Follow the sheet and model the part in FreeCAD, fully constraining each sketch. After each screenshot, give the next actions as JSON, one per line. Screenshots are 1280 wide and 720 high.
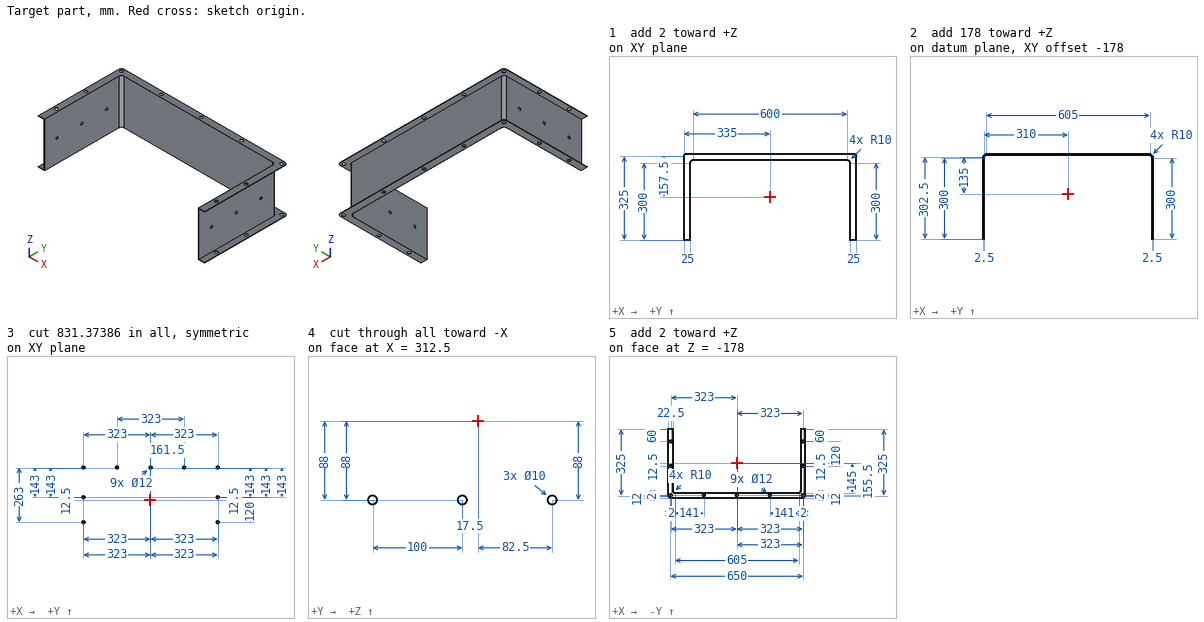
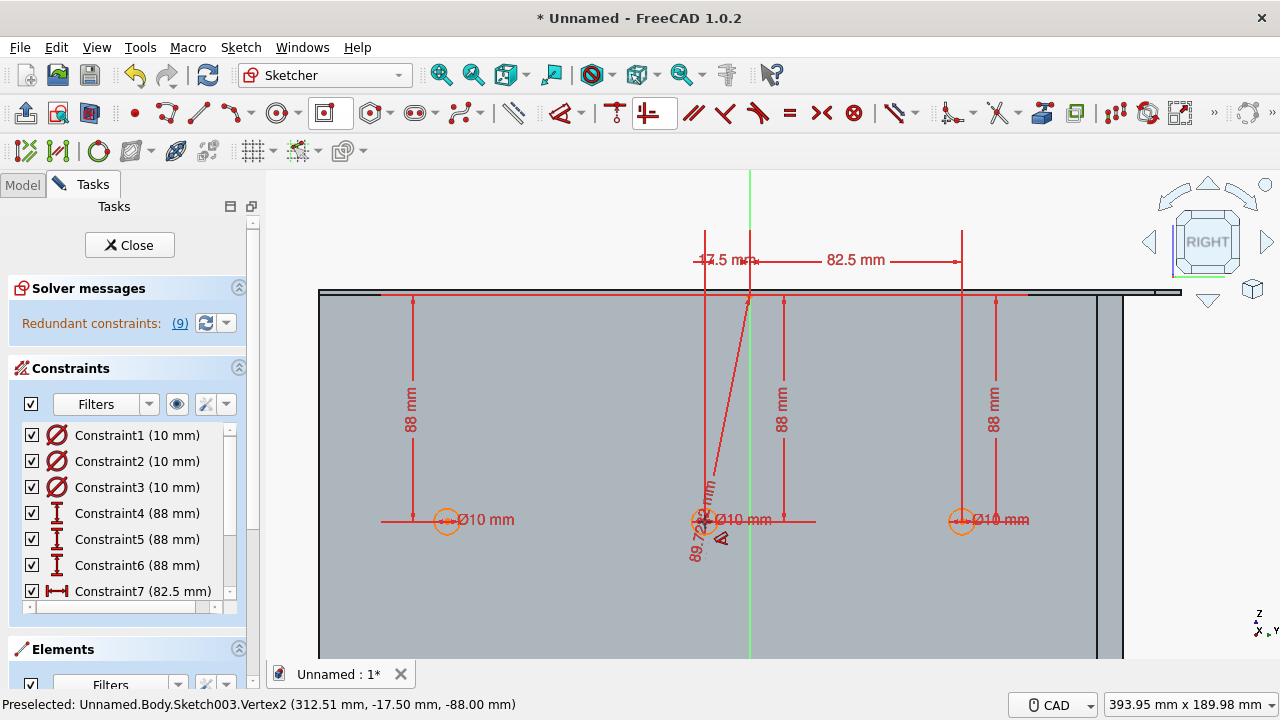
{"action": "left_click", "coordinate": [447, 522]}
{"action": "left_click", "coordinate": [576, 556]}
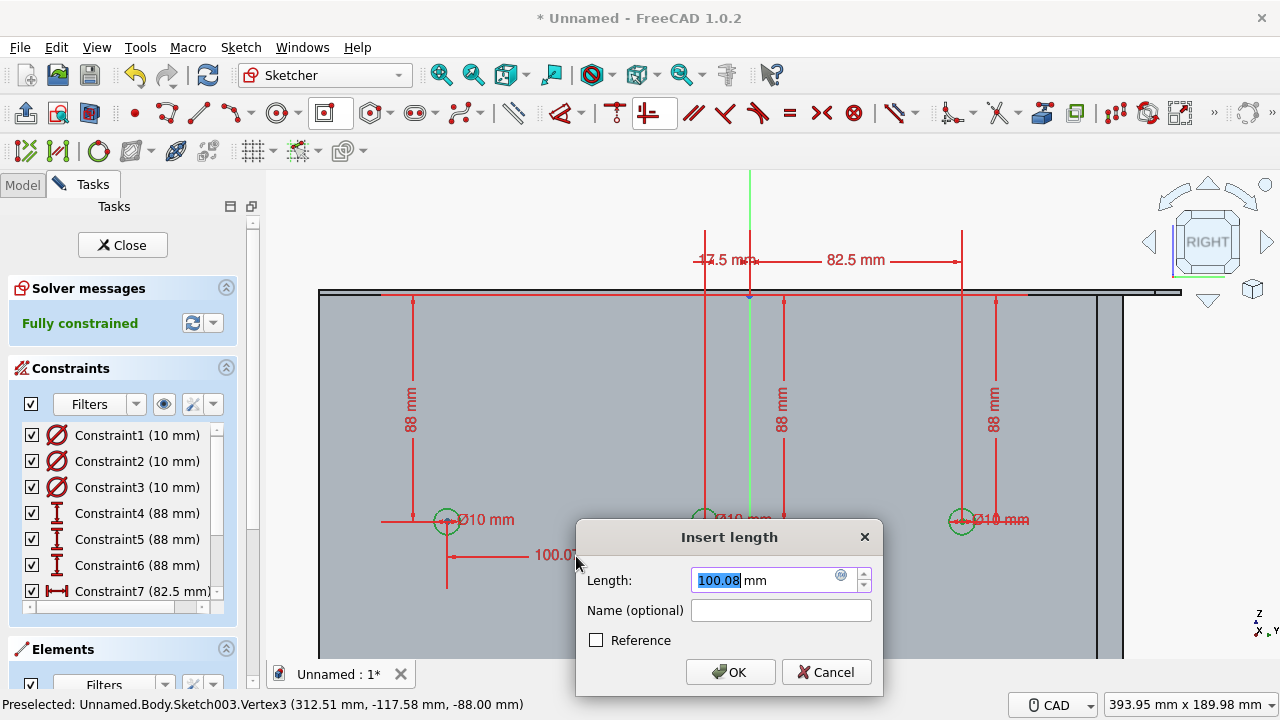
{"action": "type", "text": "100"}
{"action": "key", "text": "Return"}
{"action": "key", "text": "Escape"}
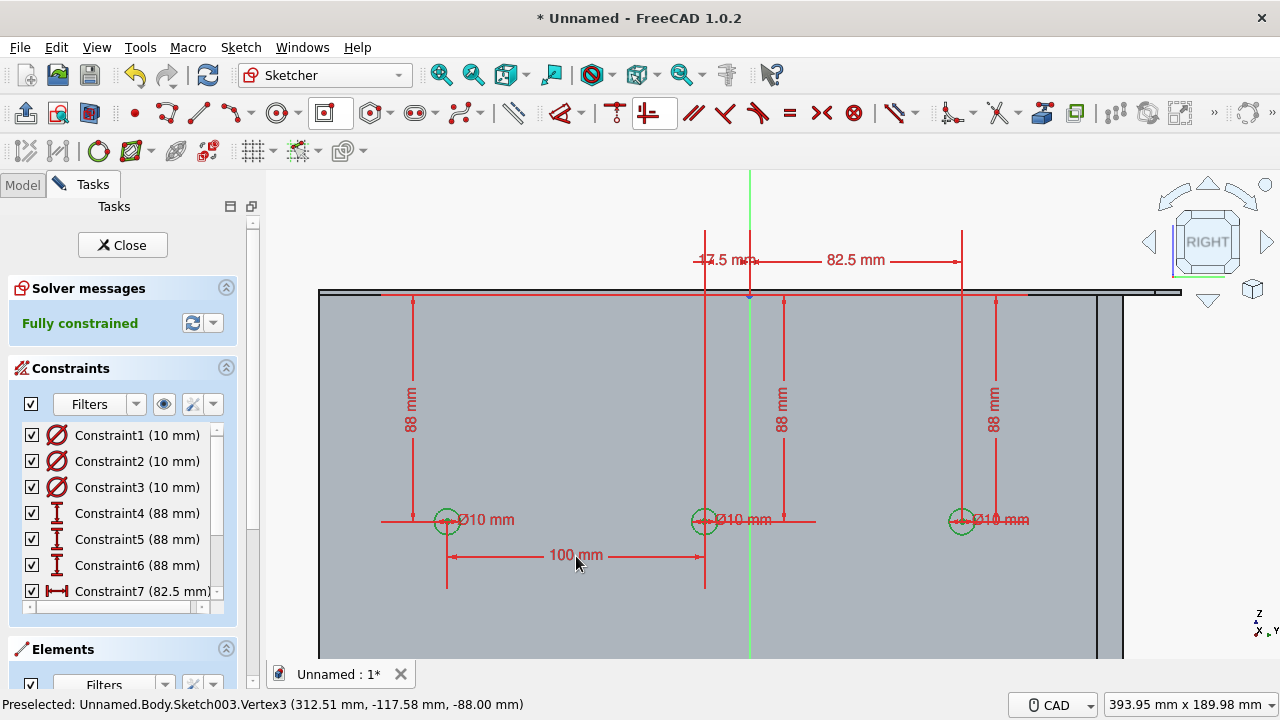
{"action": "left_click", "coordinate": [123, 245]}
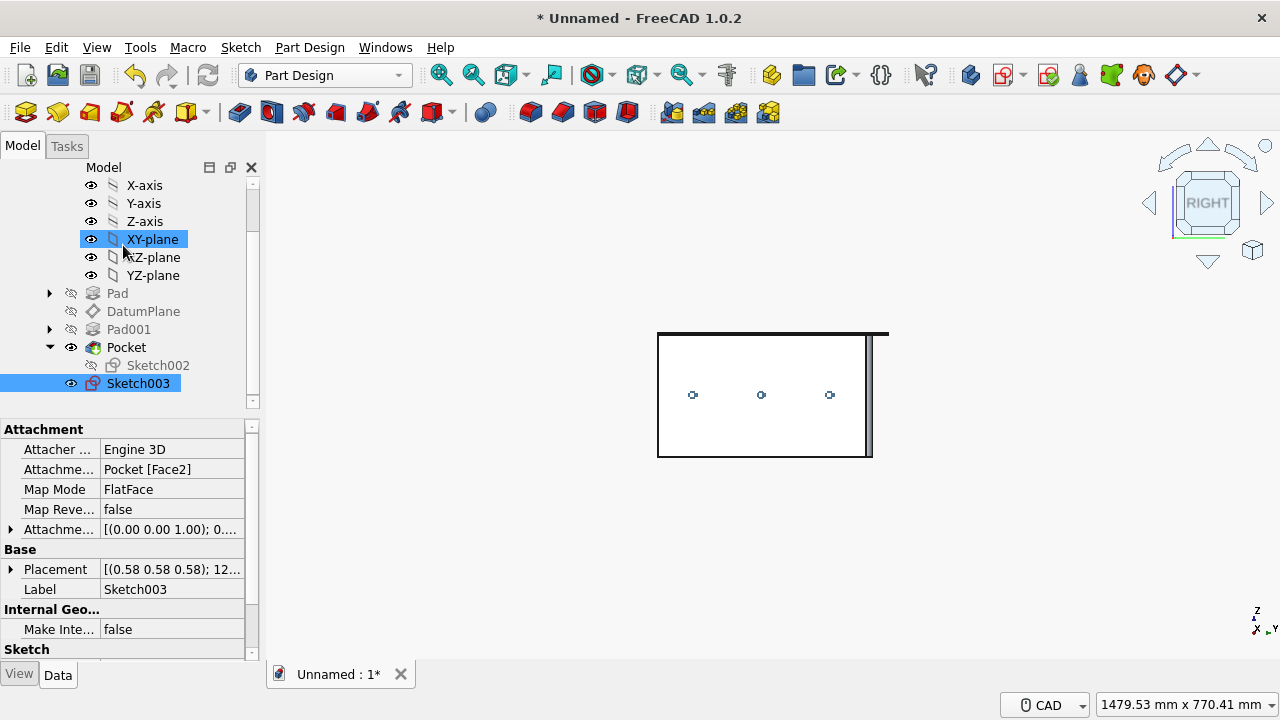
{"action": "left_click", "coordinate": [240, 112]}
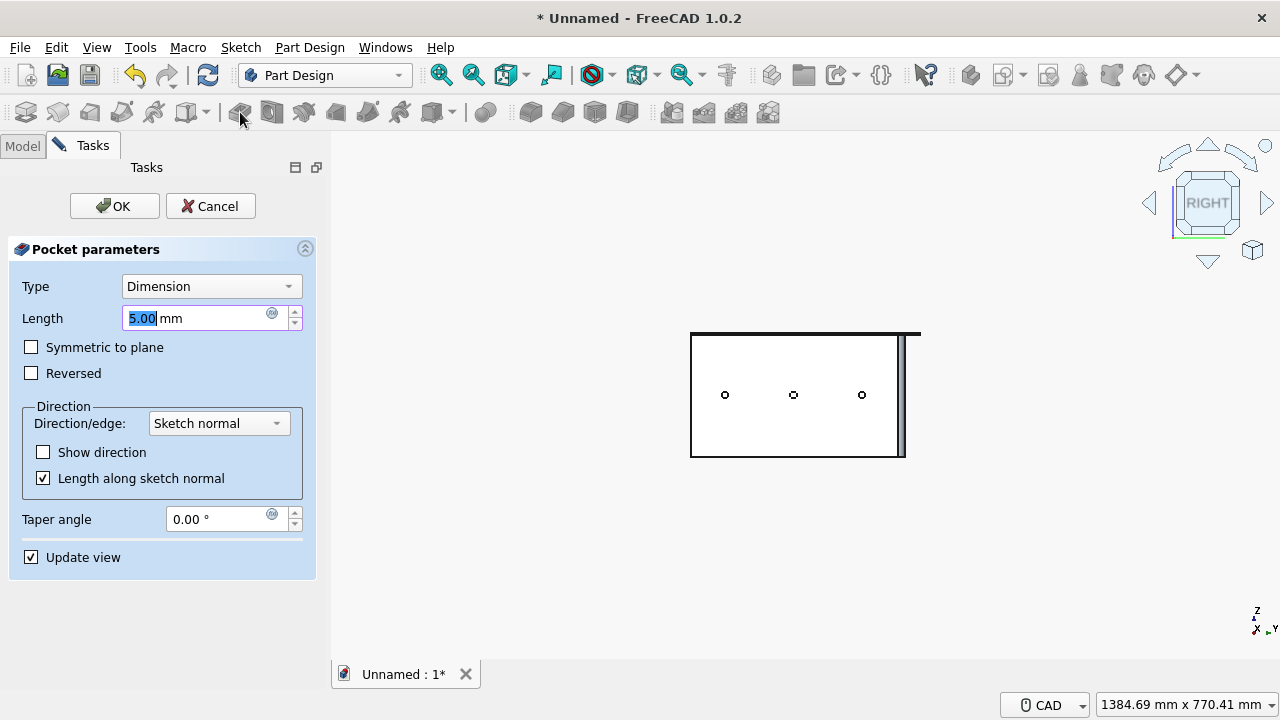
{"action": "left_click", "coordinate": [212, 286]}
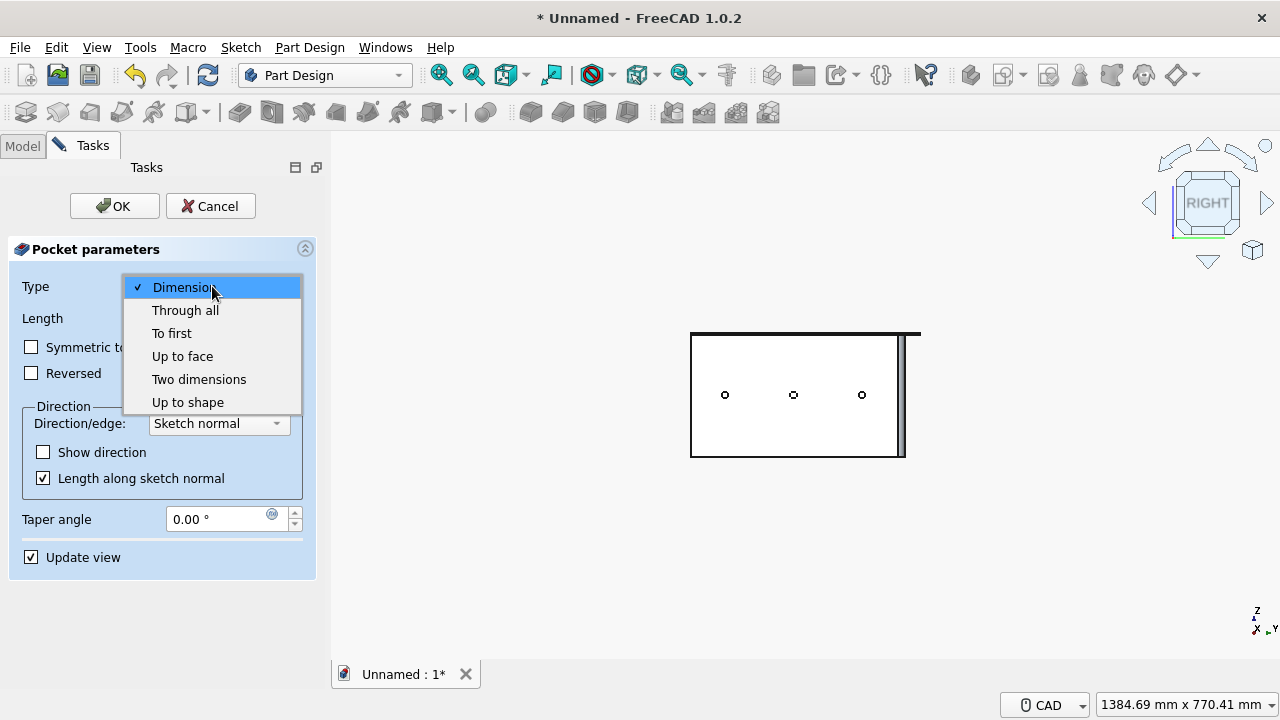
{"action": "left_click", "coordinate": [212, 310]}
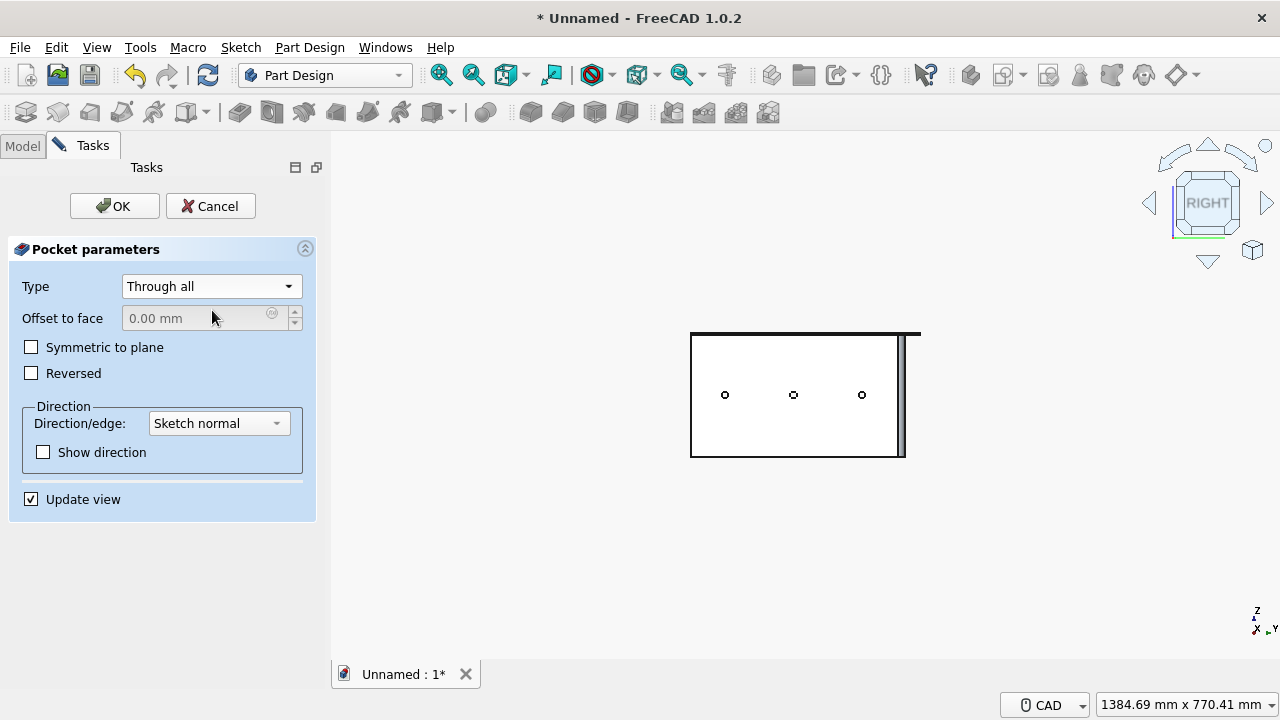
{"action": "left_click", "coordinate": [115, 206]}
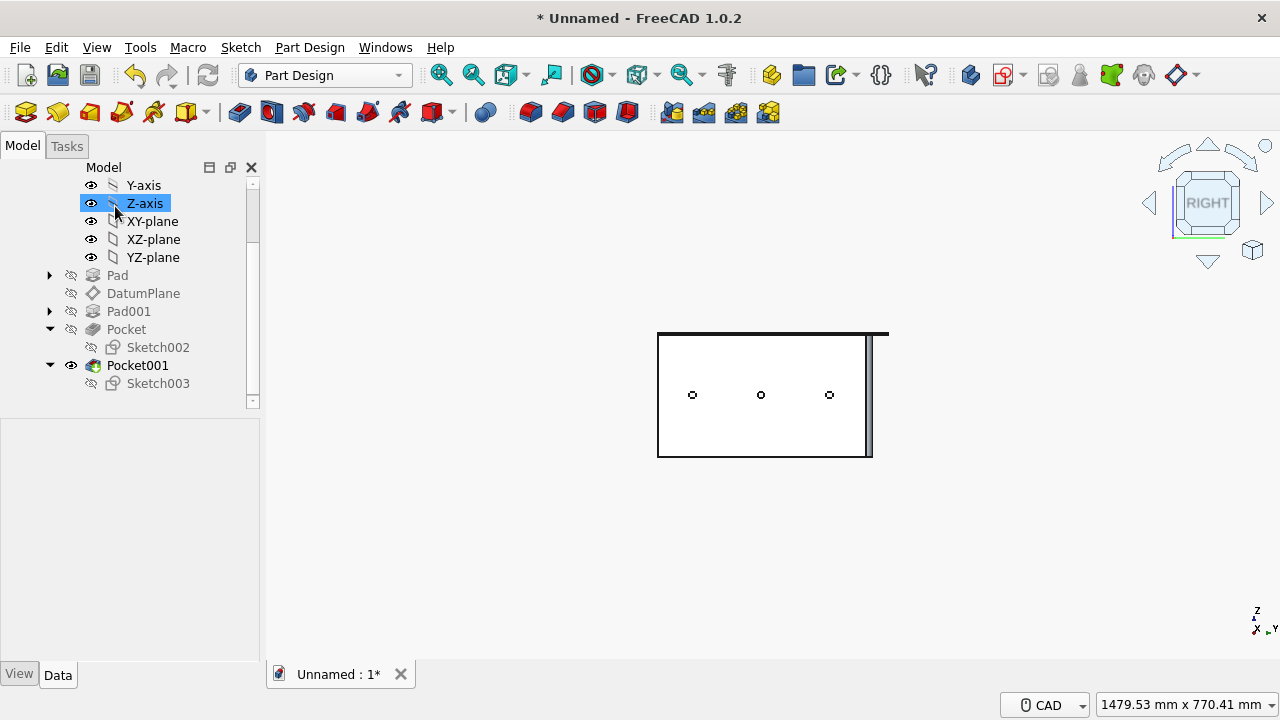
{"action": "left_click", "coordinate": [442, 76]}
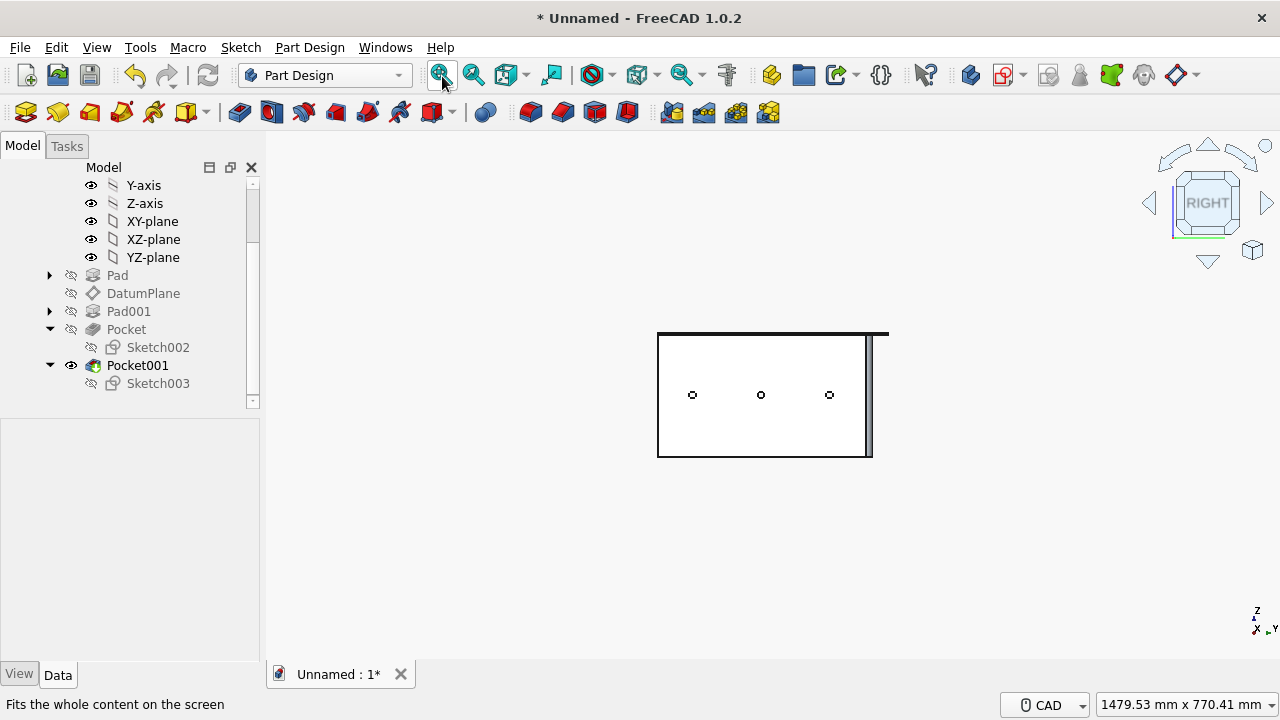
{"action": "key", "text": "5"}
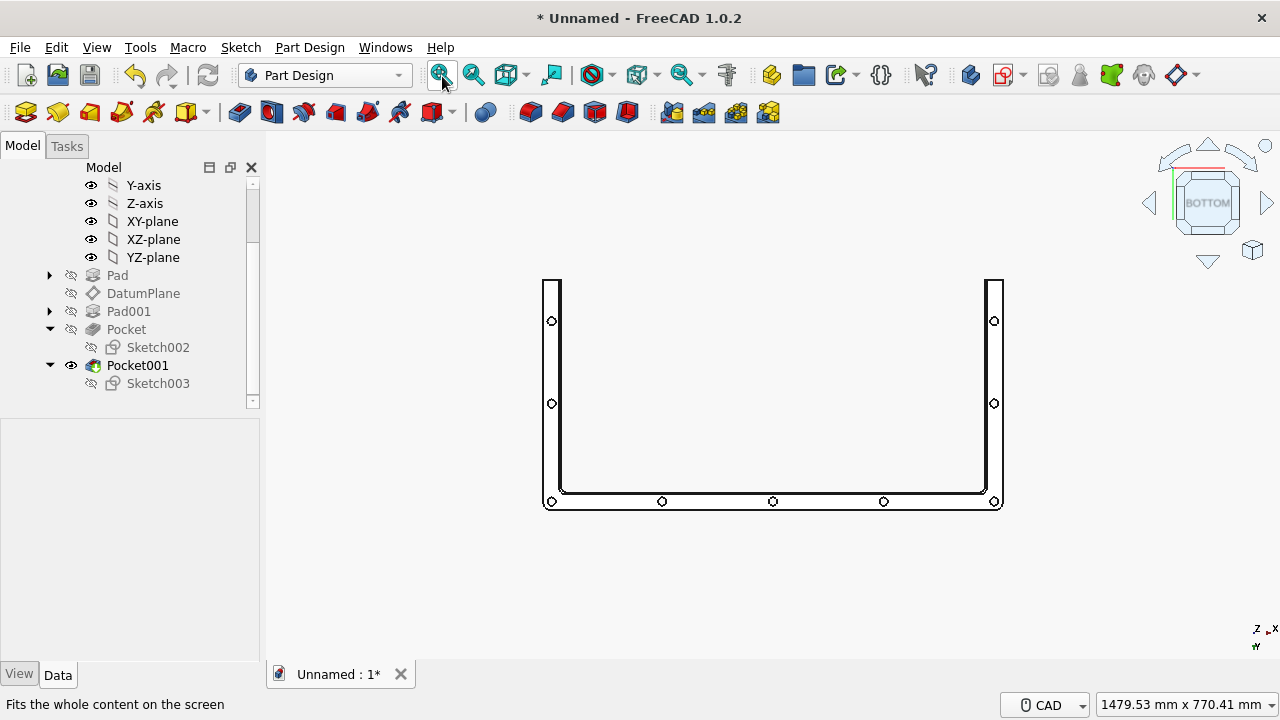
{"action": "scroll", "coordinate": [984, 491], "scroll_direction": "up", "scroll_amount": 14}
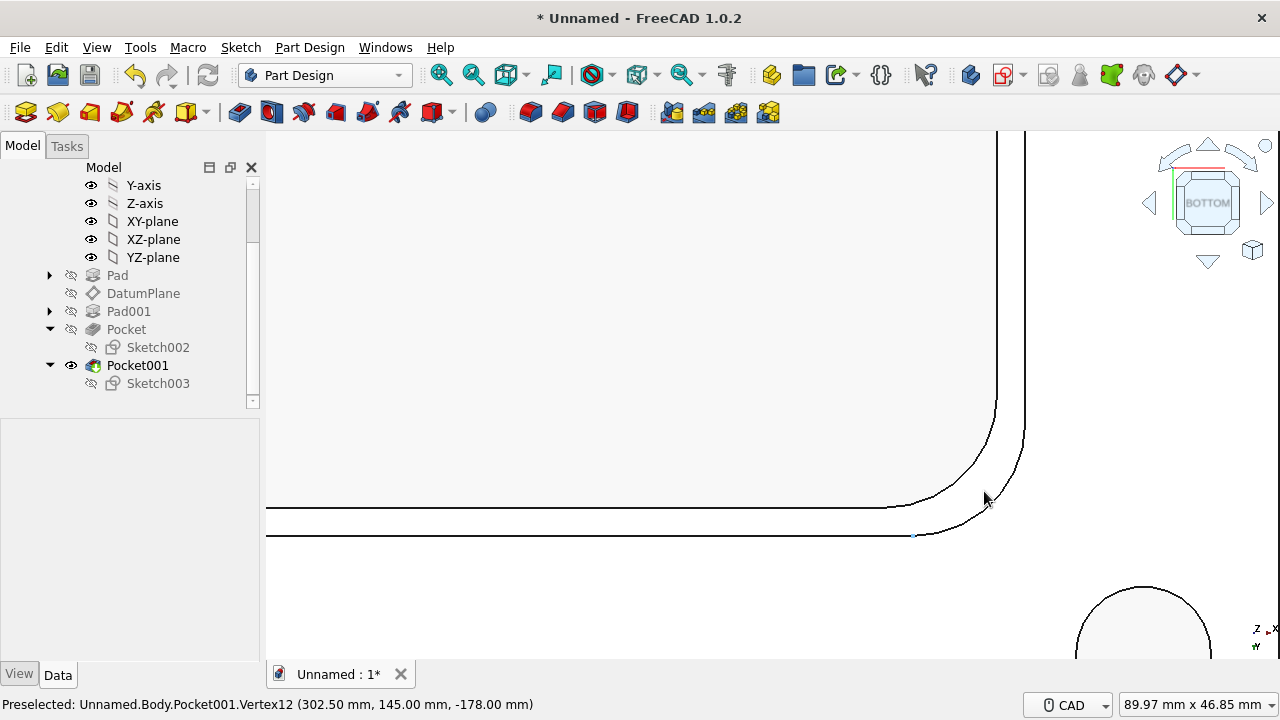
{"action": "left_click", "coordinate": [980, 495]}